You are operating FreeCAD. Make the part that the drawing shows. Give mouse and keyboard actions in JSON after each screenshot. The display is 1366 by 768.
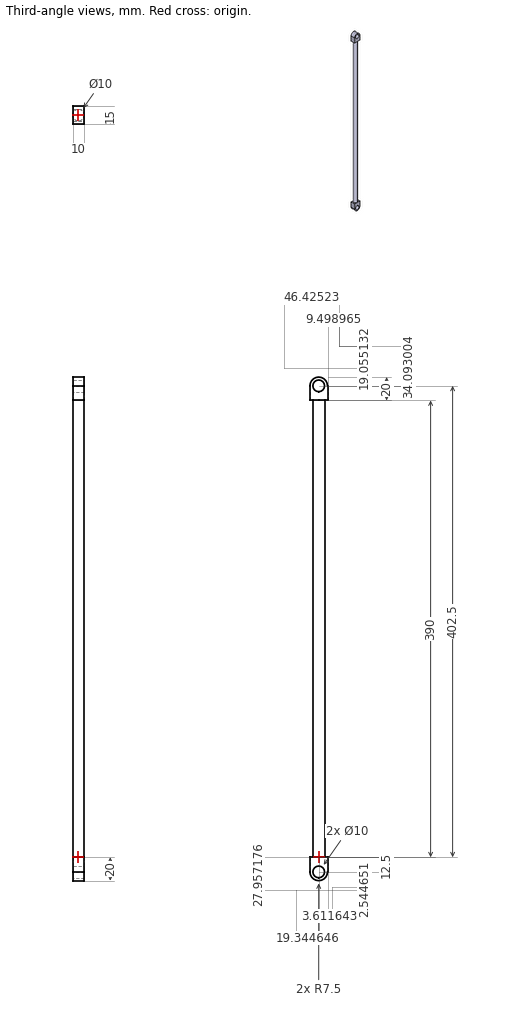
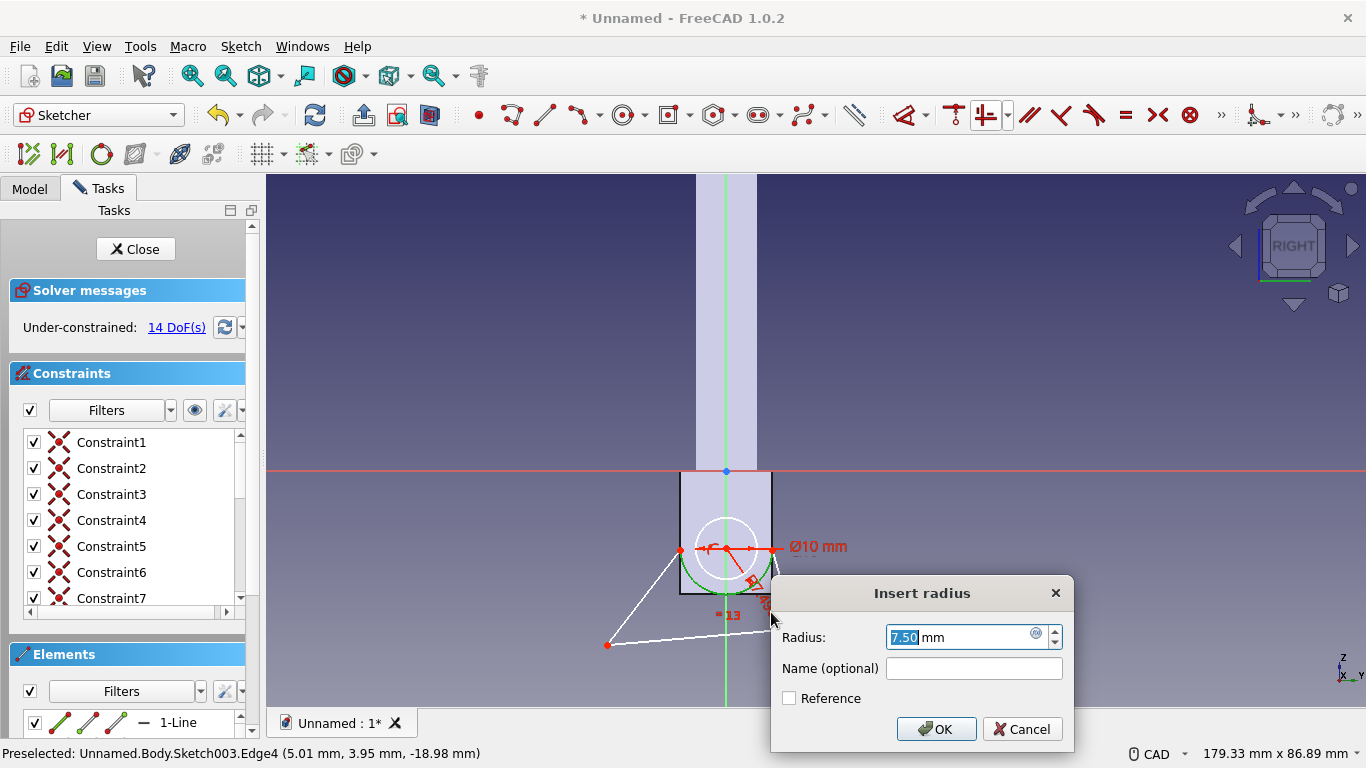
{"action": "type", "text": "7.5"}
{"action": "key", "text": "Return"}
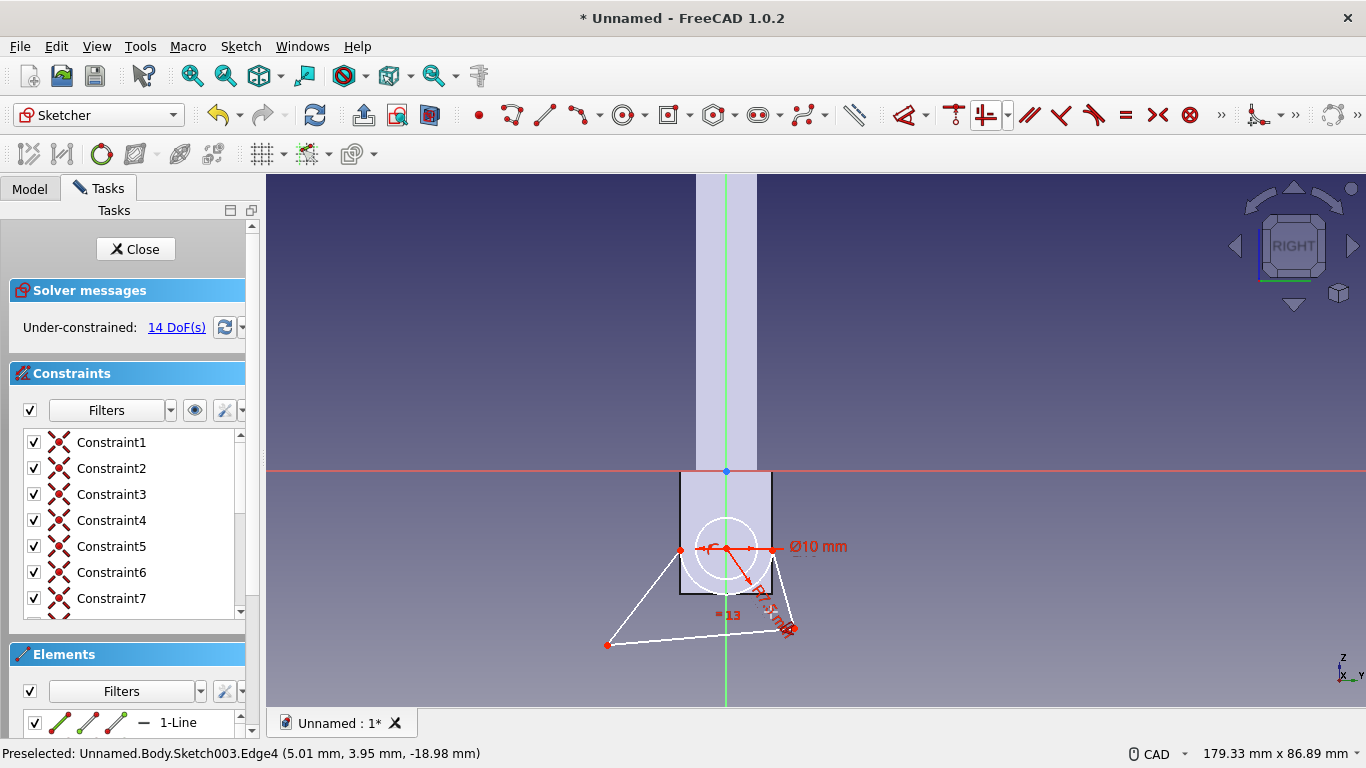
{"action": "left_click", "coordinate": [726, 549]}
{"action": "left_click", "coordinate": [760, 510]}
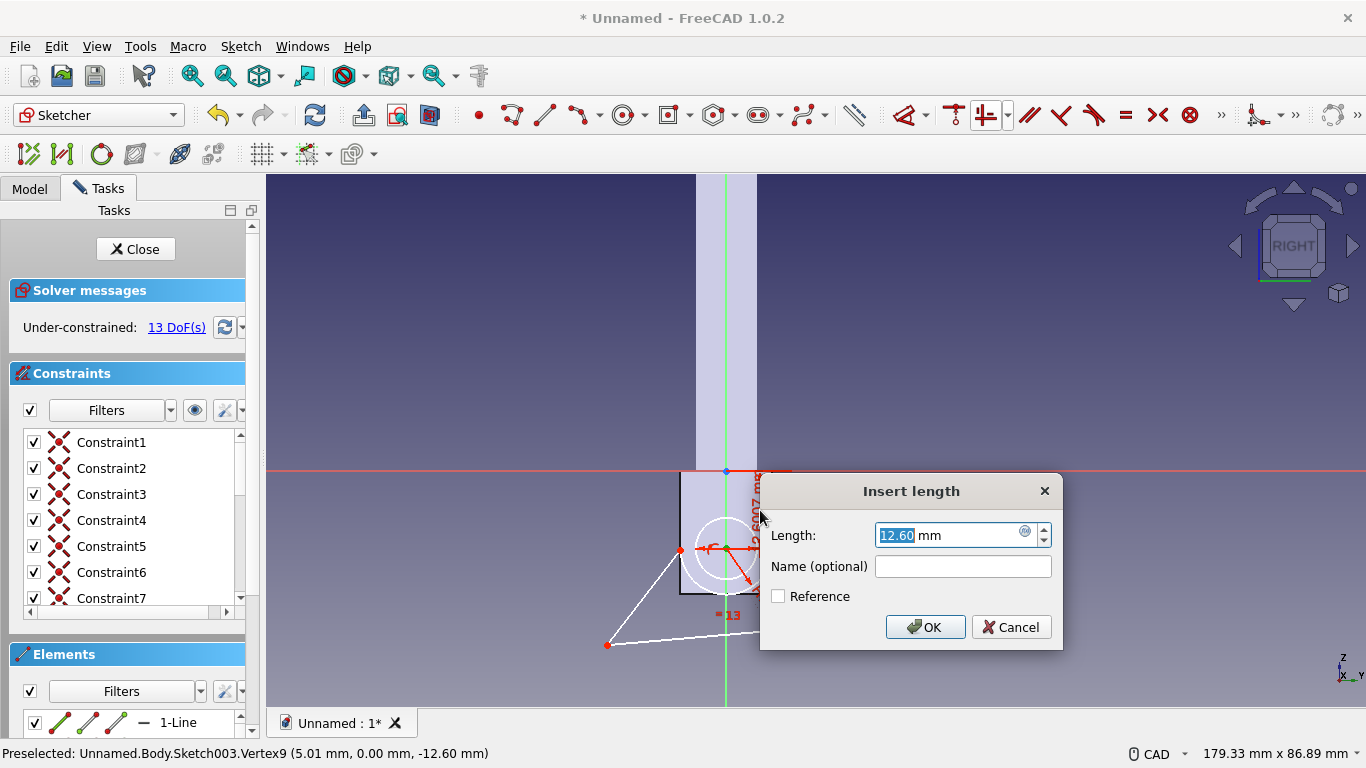
{"action": "type", "text": "12.5"}
{"action": "key", "text": "Return"}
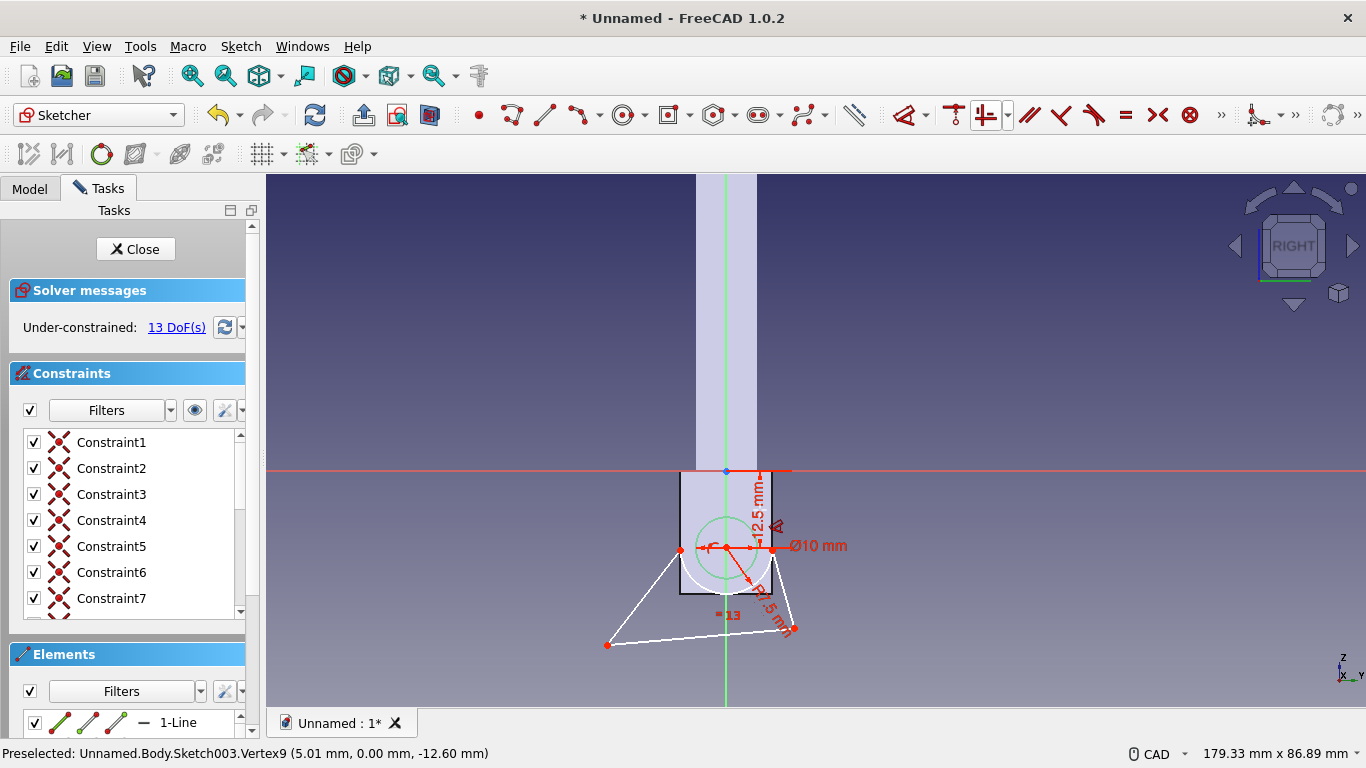
{"action": "left_click", "coordinate": [681, 550]}
{"action": "left_click", "coordinate": [647, 511]}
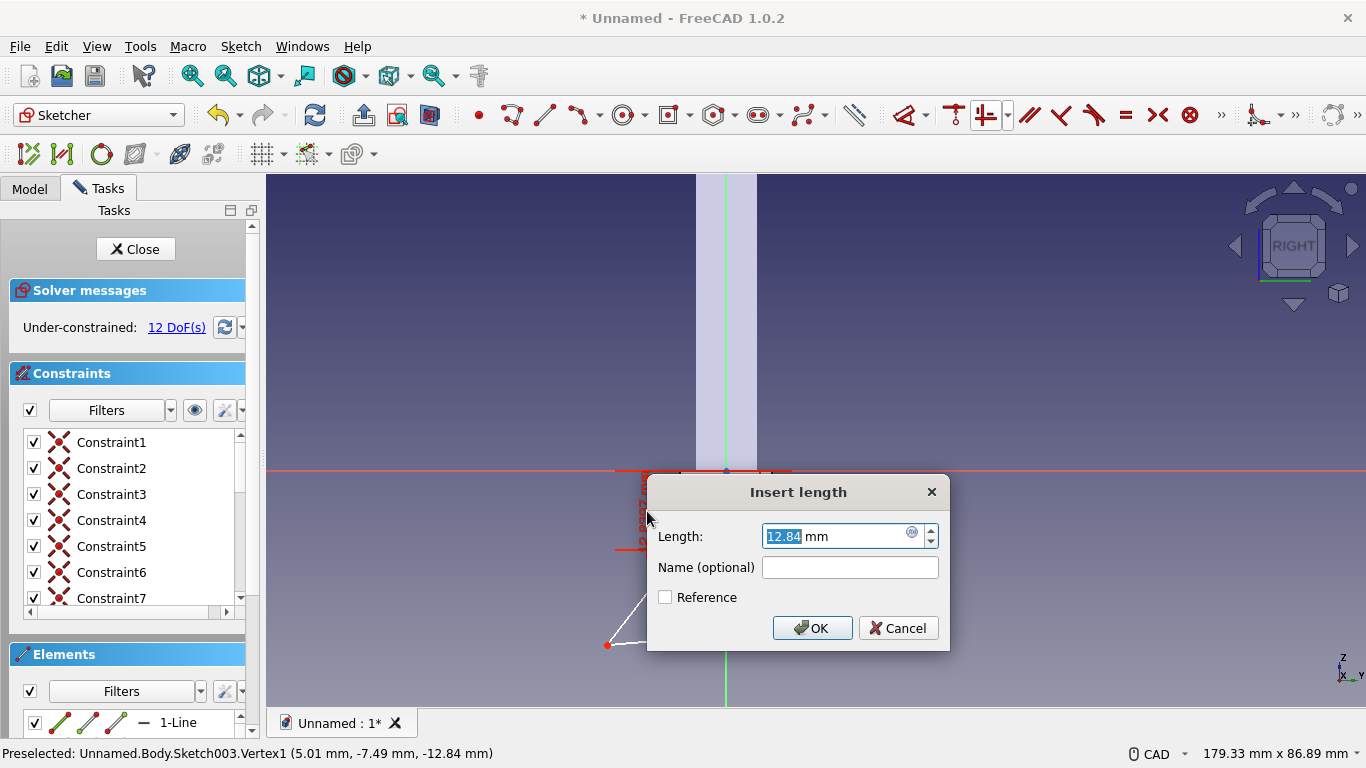
{"action": "type", "text": "12.5"}
{"action": "key", "text": "Return"}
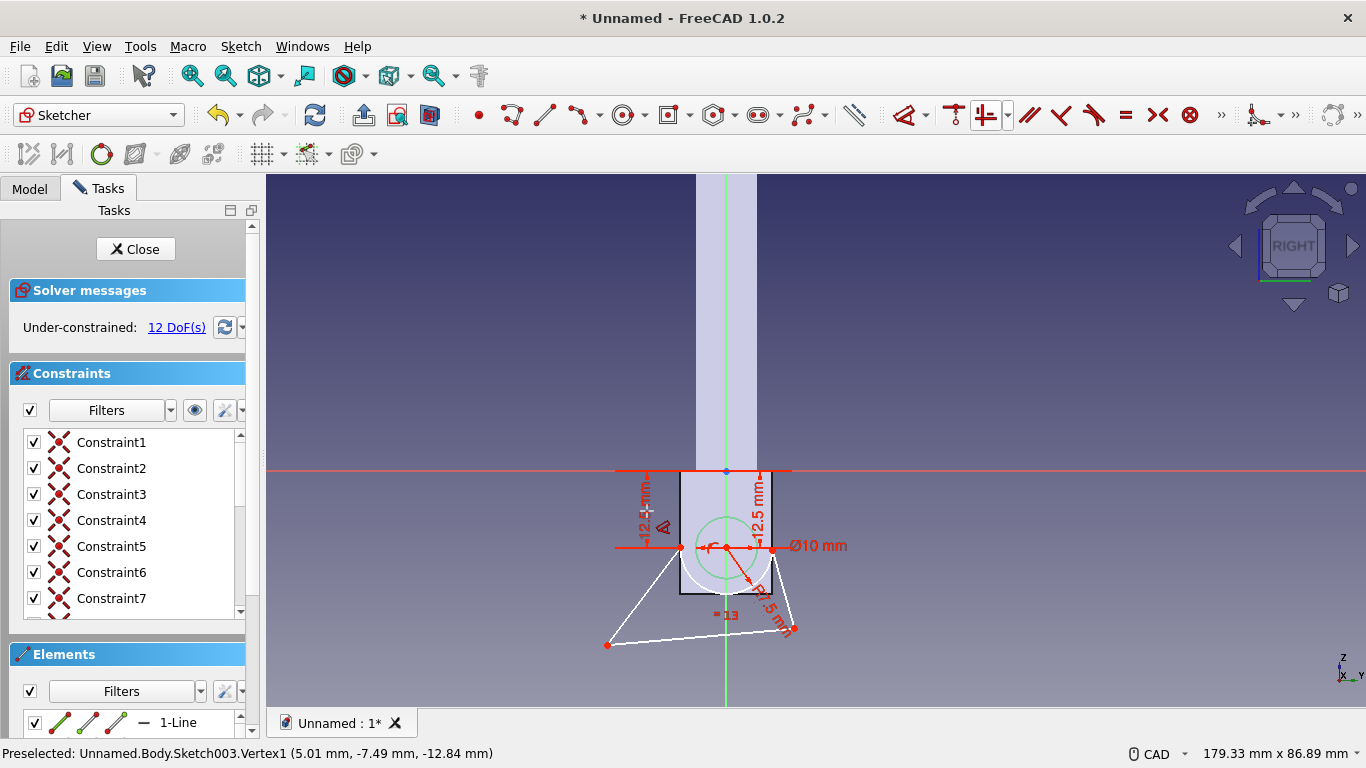
{"action": "left_click", "coordinate": [772, 550]}
{"action": "left_click", "coordinate": [806, 538]}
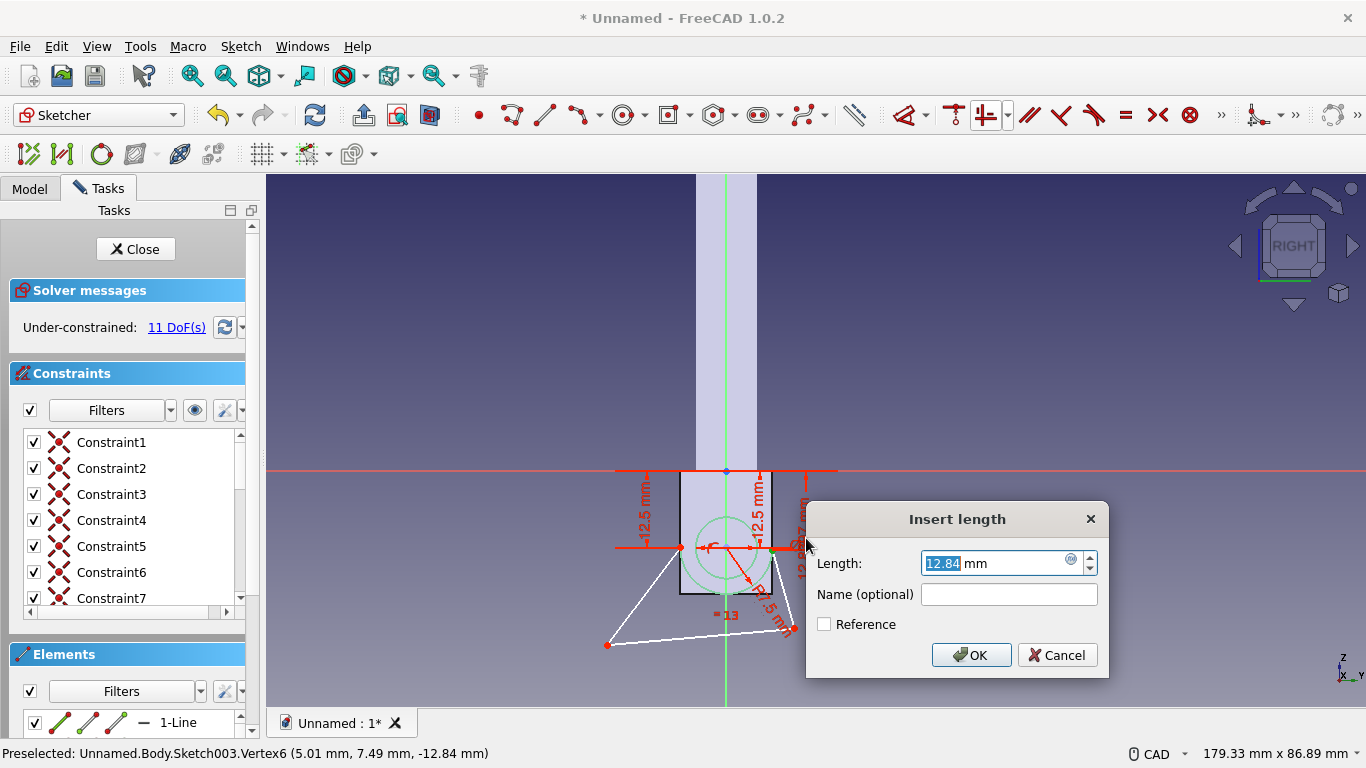
{"action": "type", "text": "12.5"}
{"action": "key", "text": "Return"}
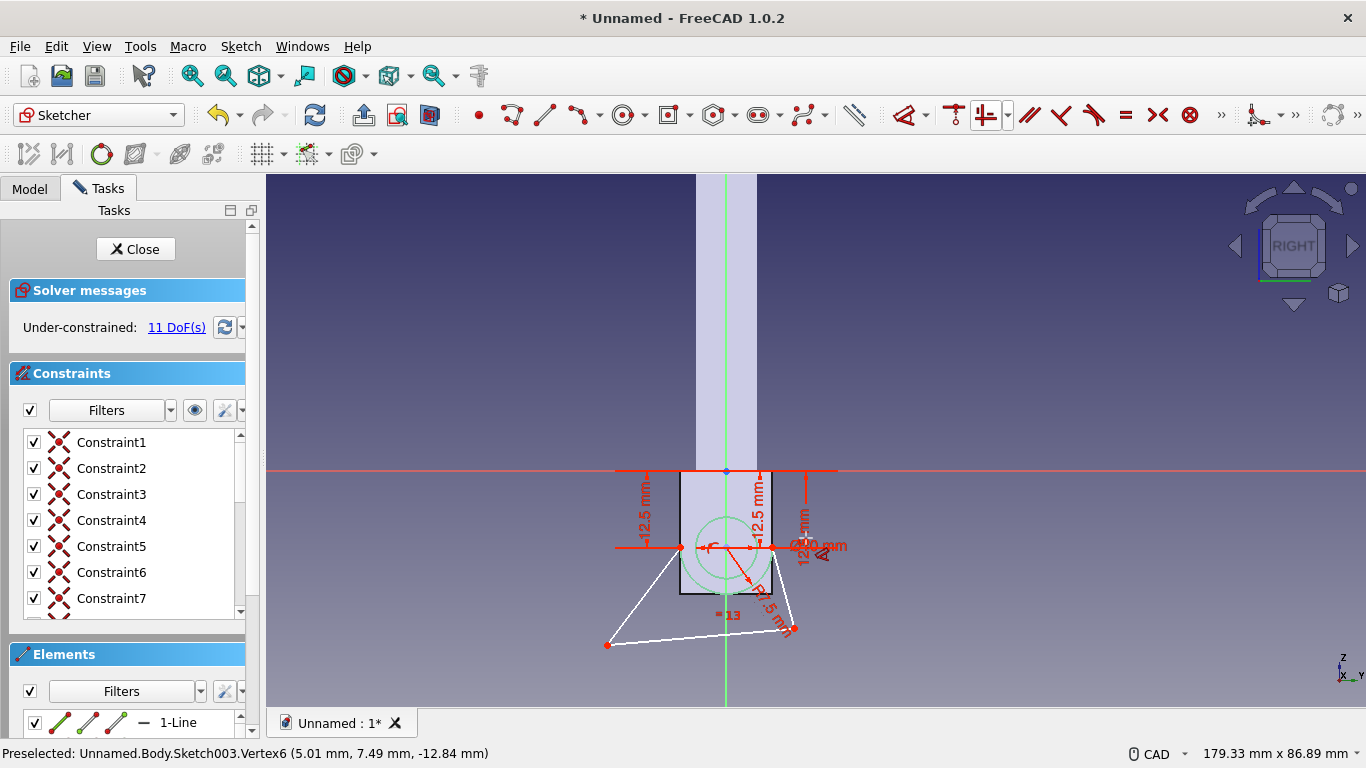
{"action": "scroll", "coordinate": [755, 593], "scroll_direction": "down", "scroll_amount": 11}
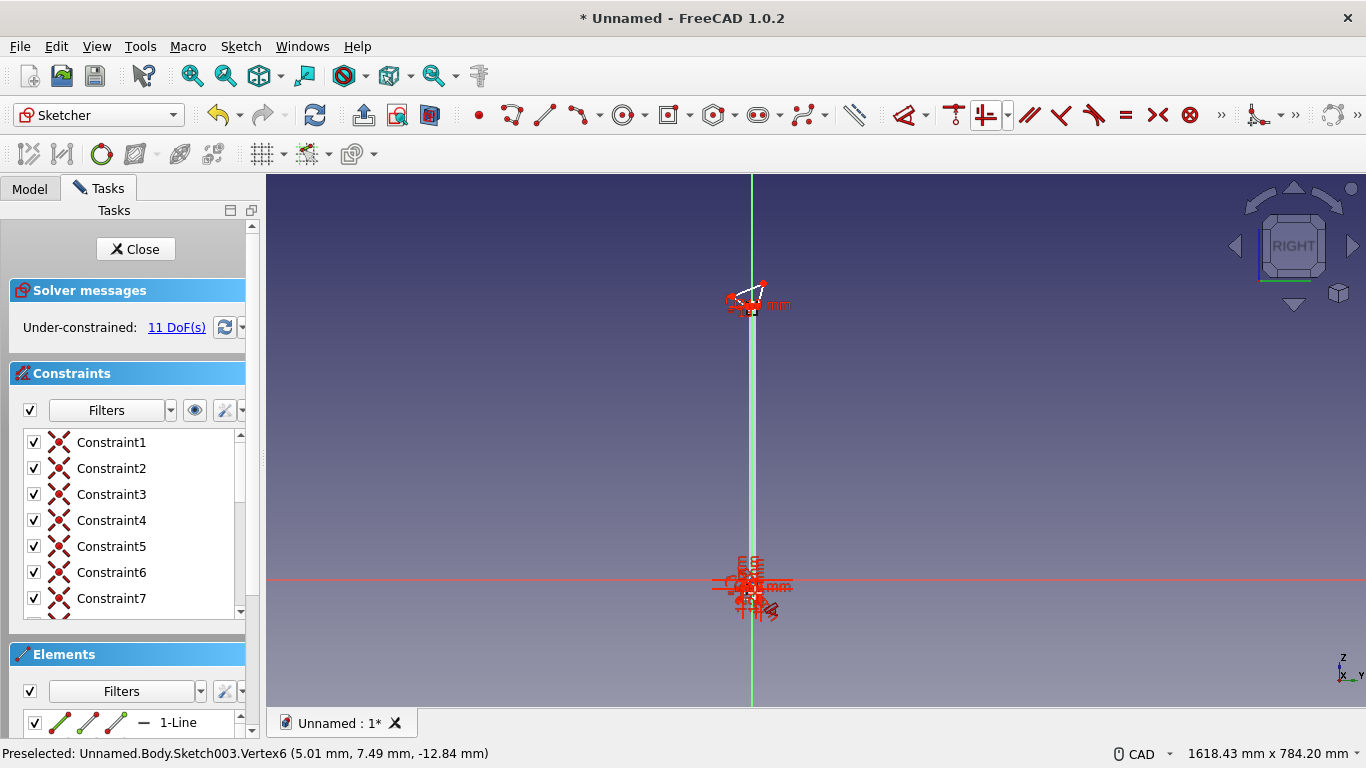
{"action": "scroll", "coordinate": [752, 307], "scroll_direction": "up", "scroll_amount": 5}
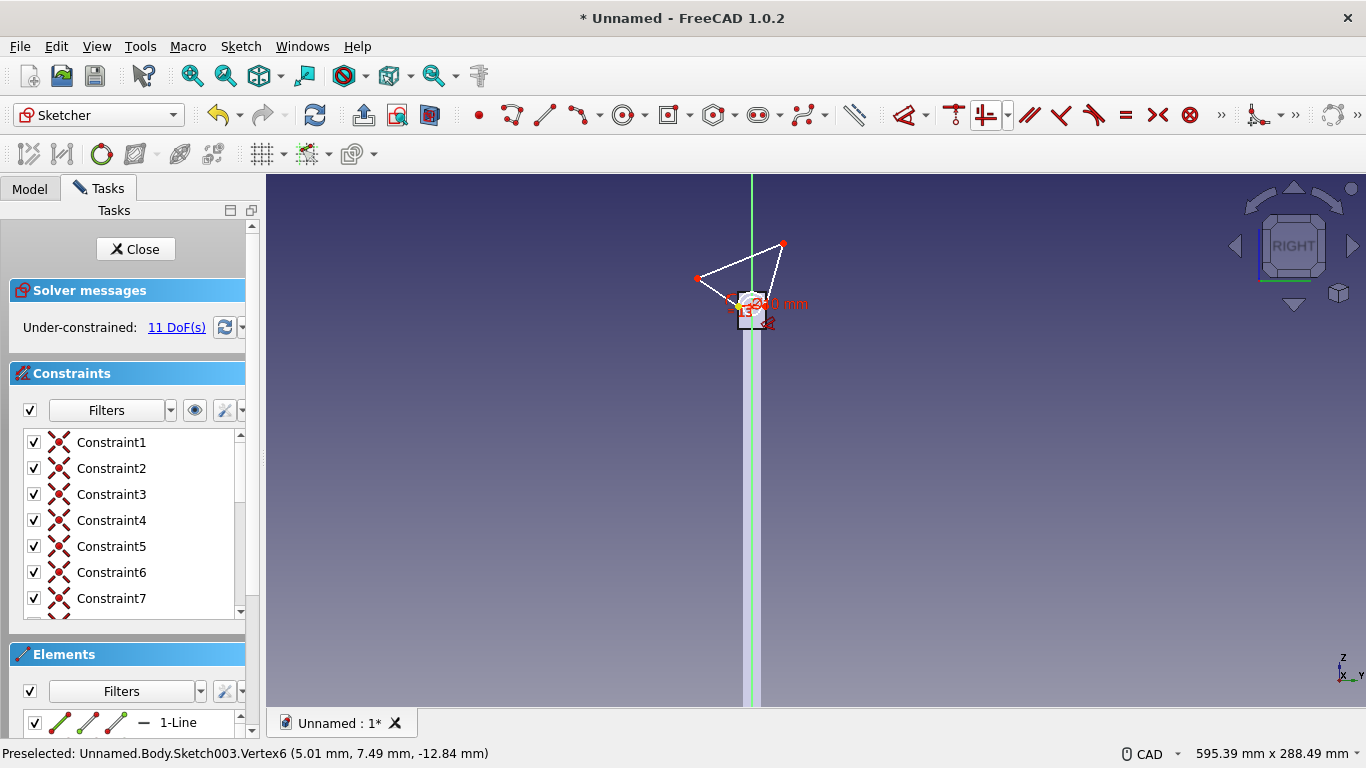
{"action": "left_click", "coordinate": [752, 306]}
{"action": "left_click", "coordinate": [786, 493]}